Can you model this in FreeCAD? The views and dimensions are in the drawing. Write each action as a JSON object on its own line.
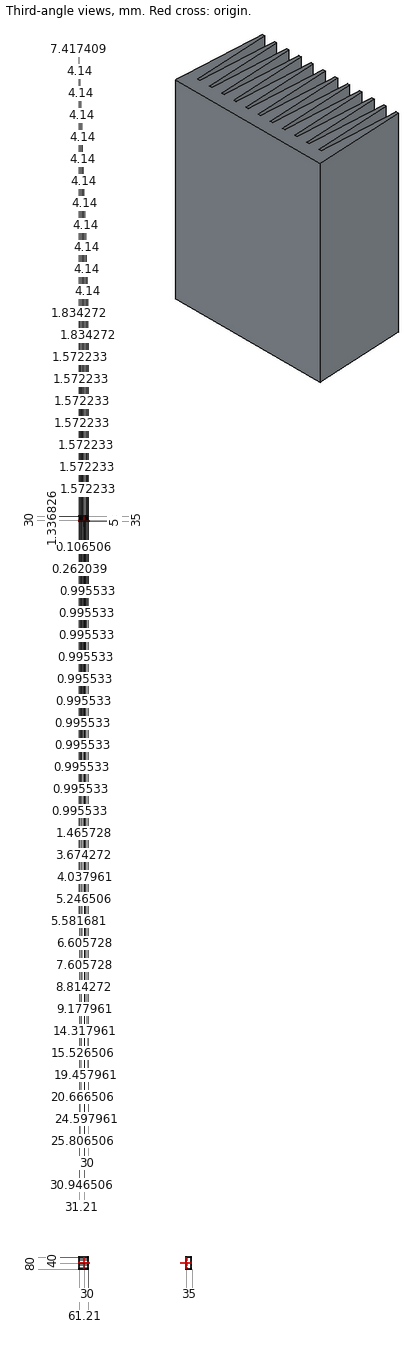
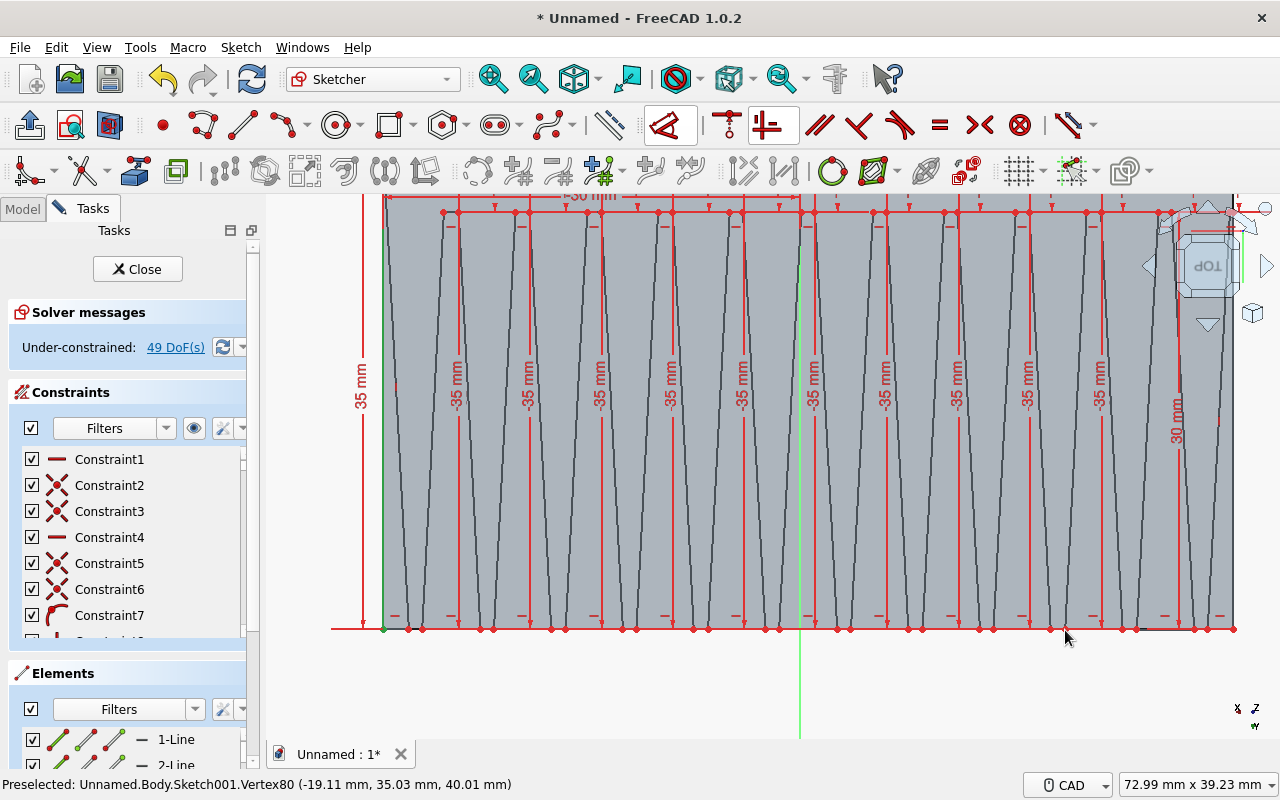
{"action": "scroll", "coordinate": [494, 630], "scroll_direction": "down", "scroll_amount": 2}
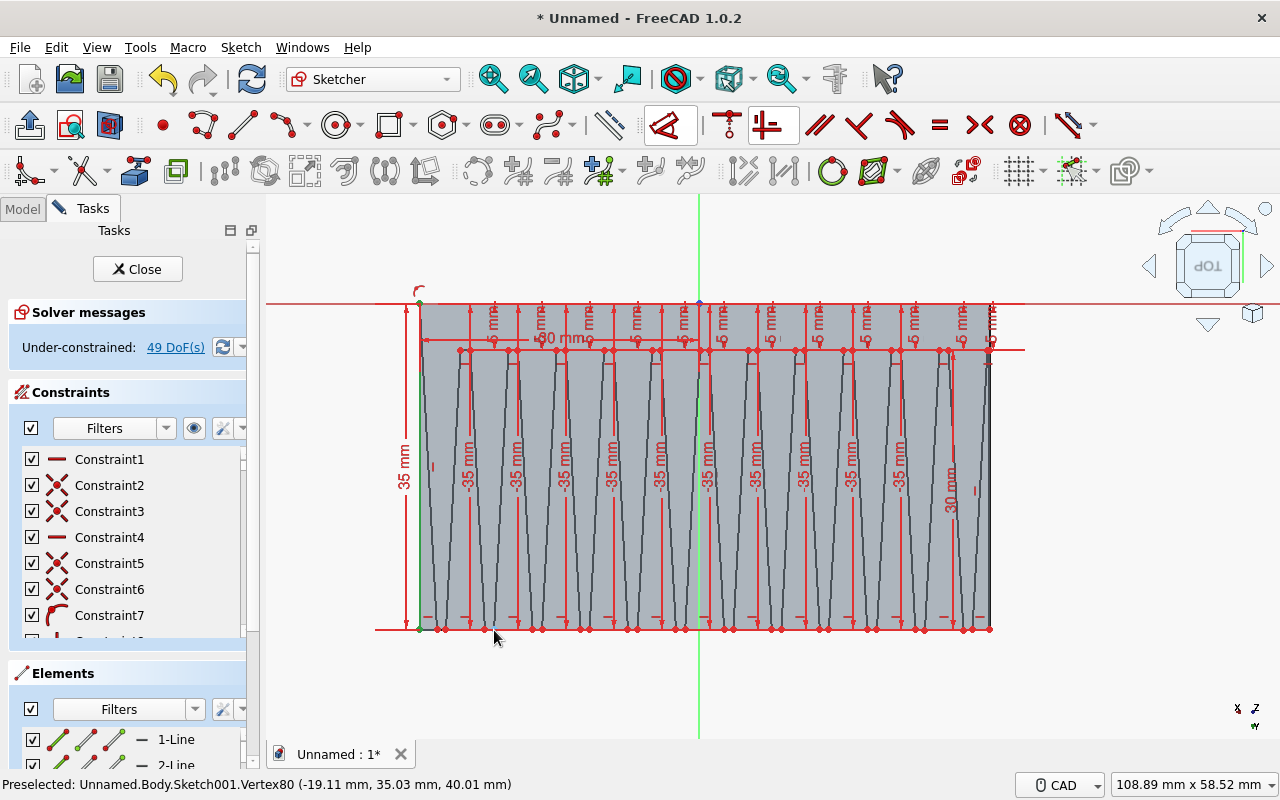
{"action": "scroll", "coordinate": [925, 630], "scroll_direction": "up", "scroll_amount": 2}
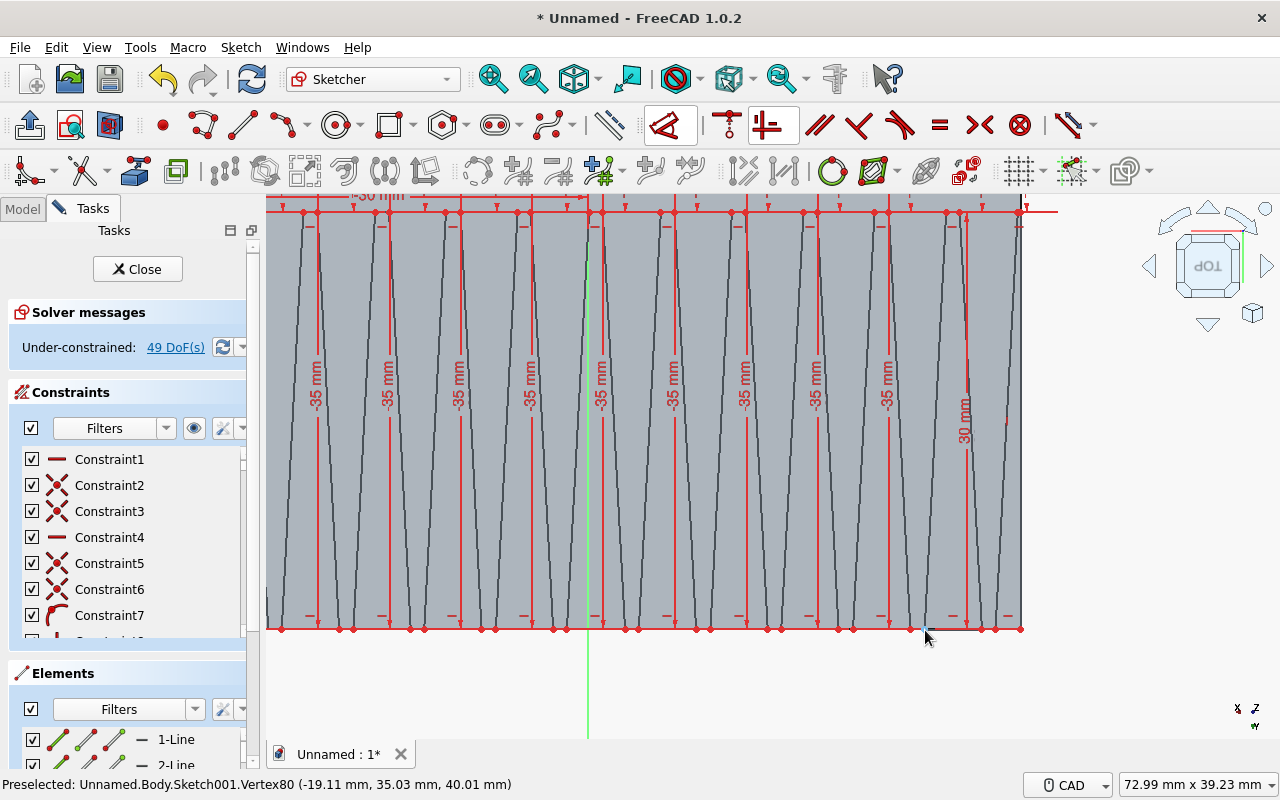
{"action": "left_click", "coordinate": [925, 630]}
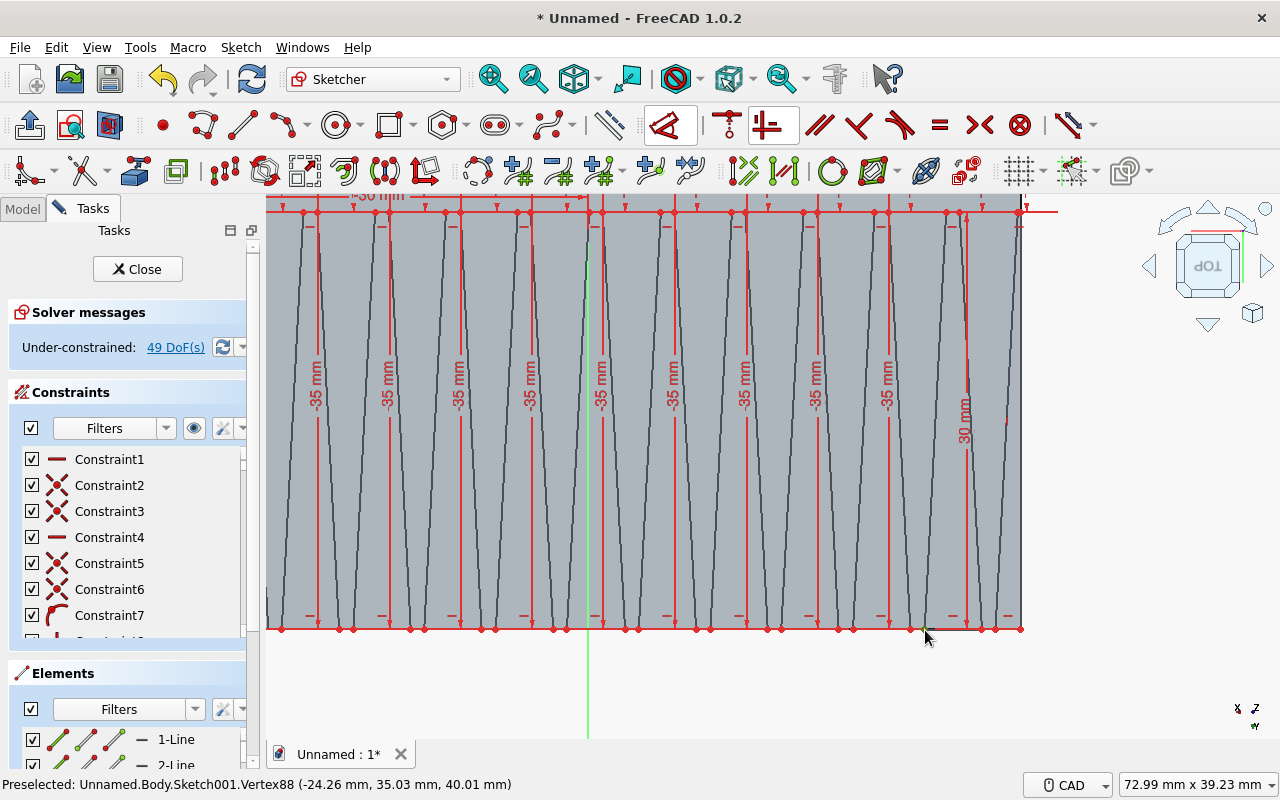
{"action": "key", "text": "i"}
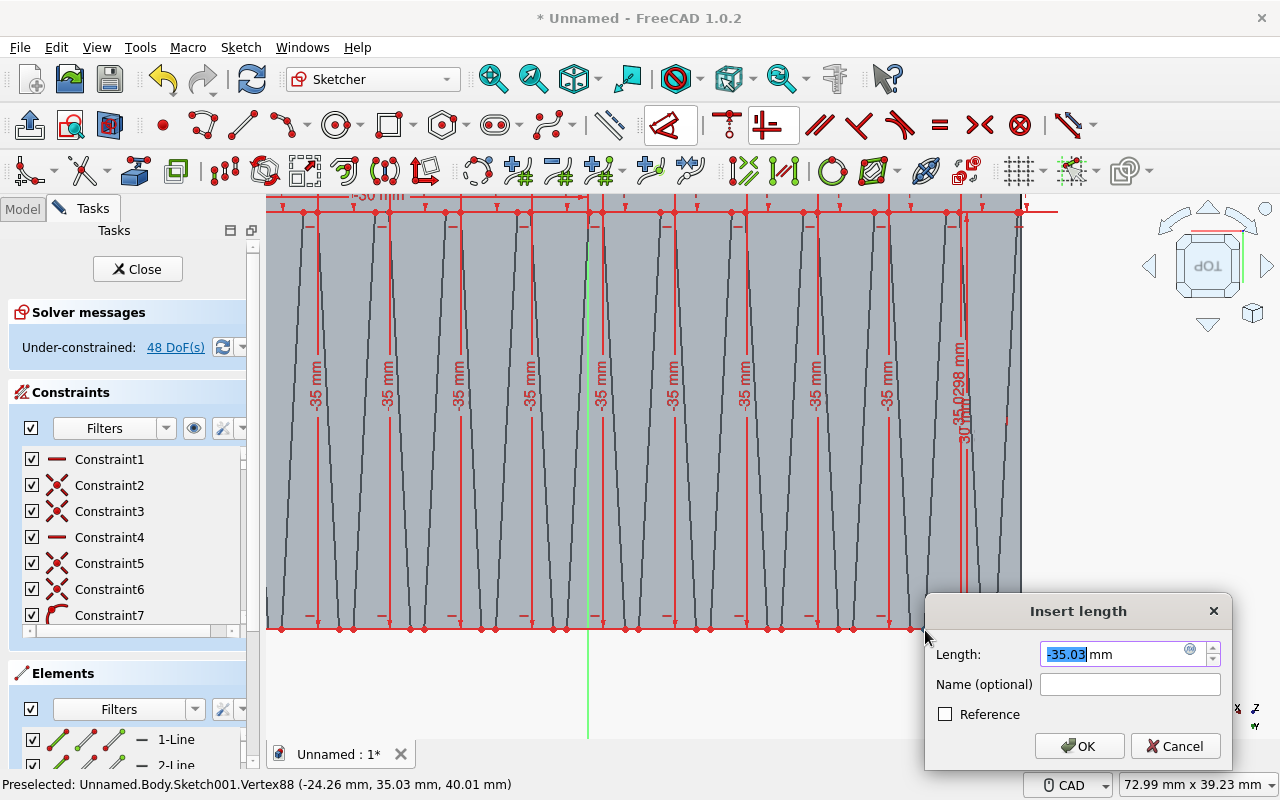
{"action": "type", "text": "-35"}
{"action": "key", "text": "Return"}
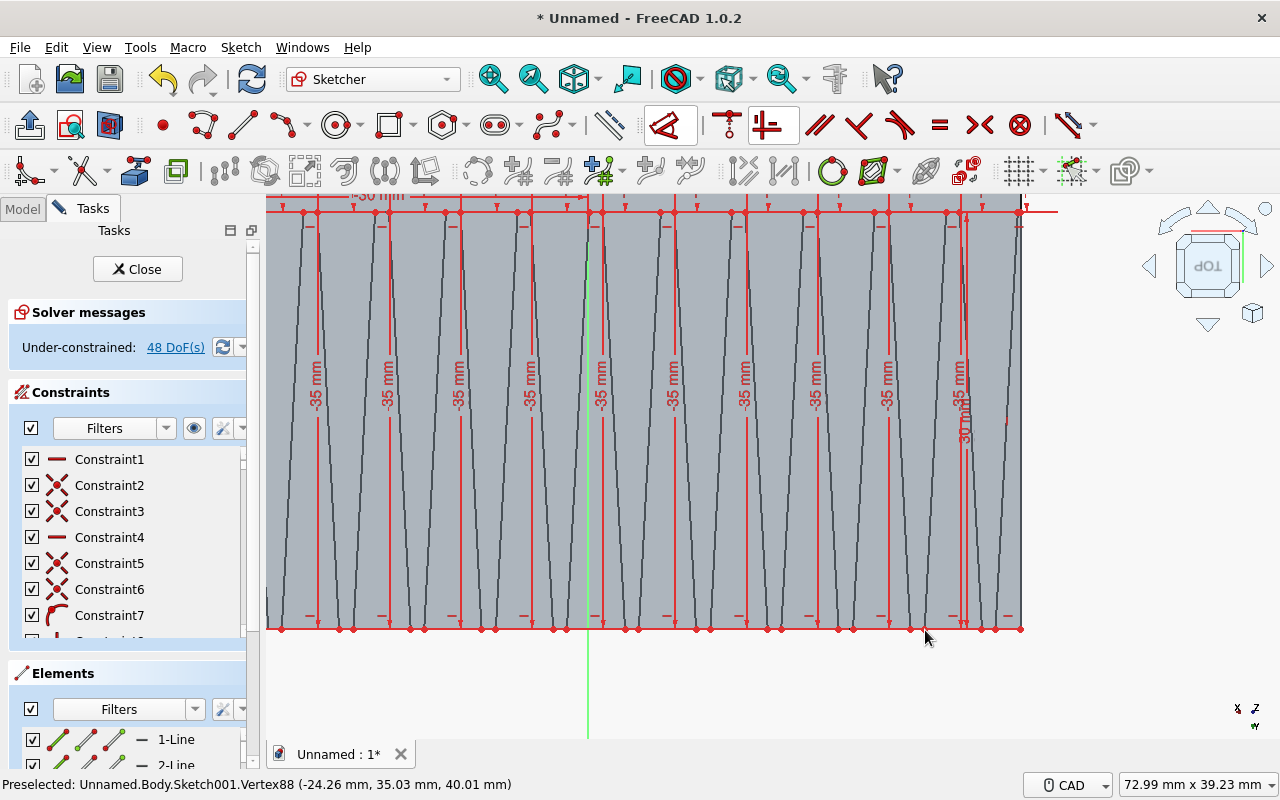
{"action": "scroll", "coordinate": [925, 630], "scroll_direction": "down", "scroll_amount": 2}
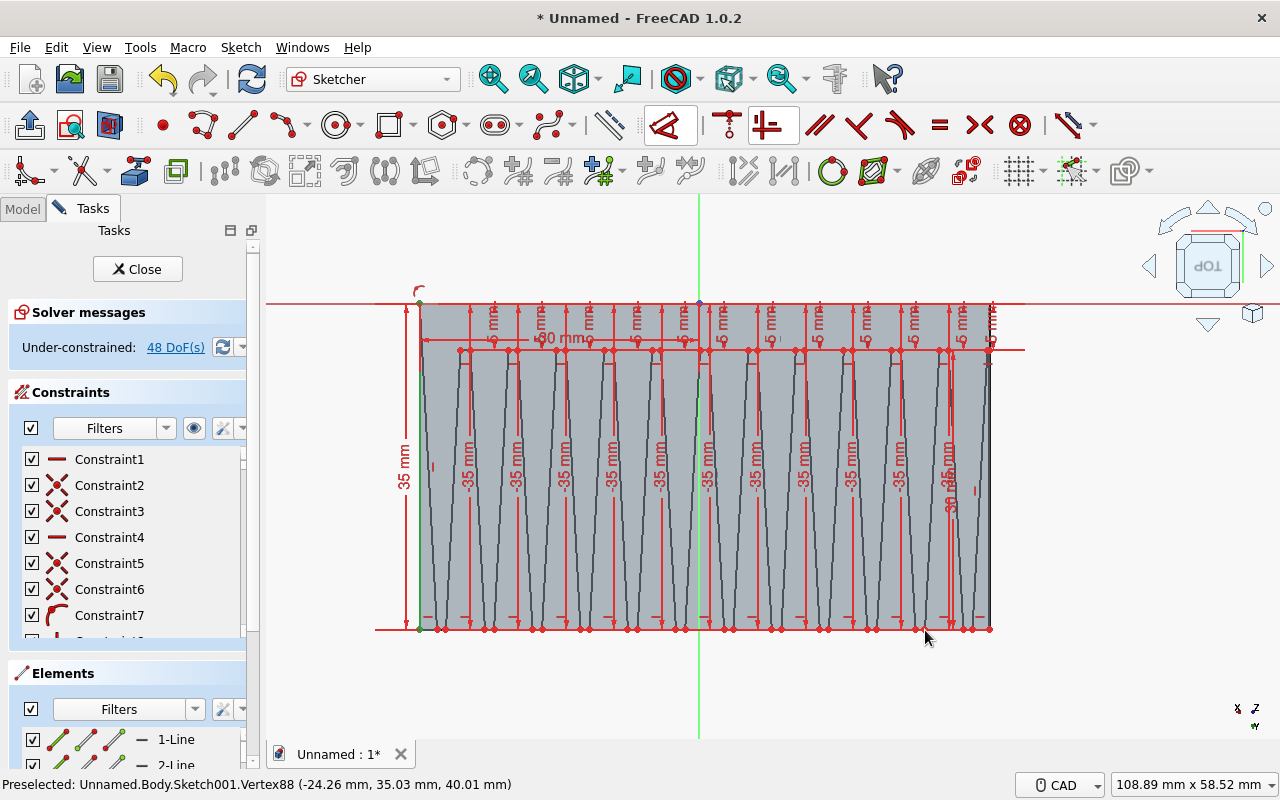
{"action": "left_click", "coordinate": [458, 630]}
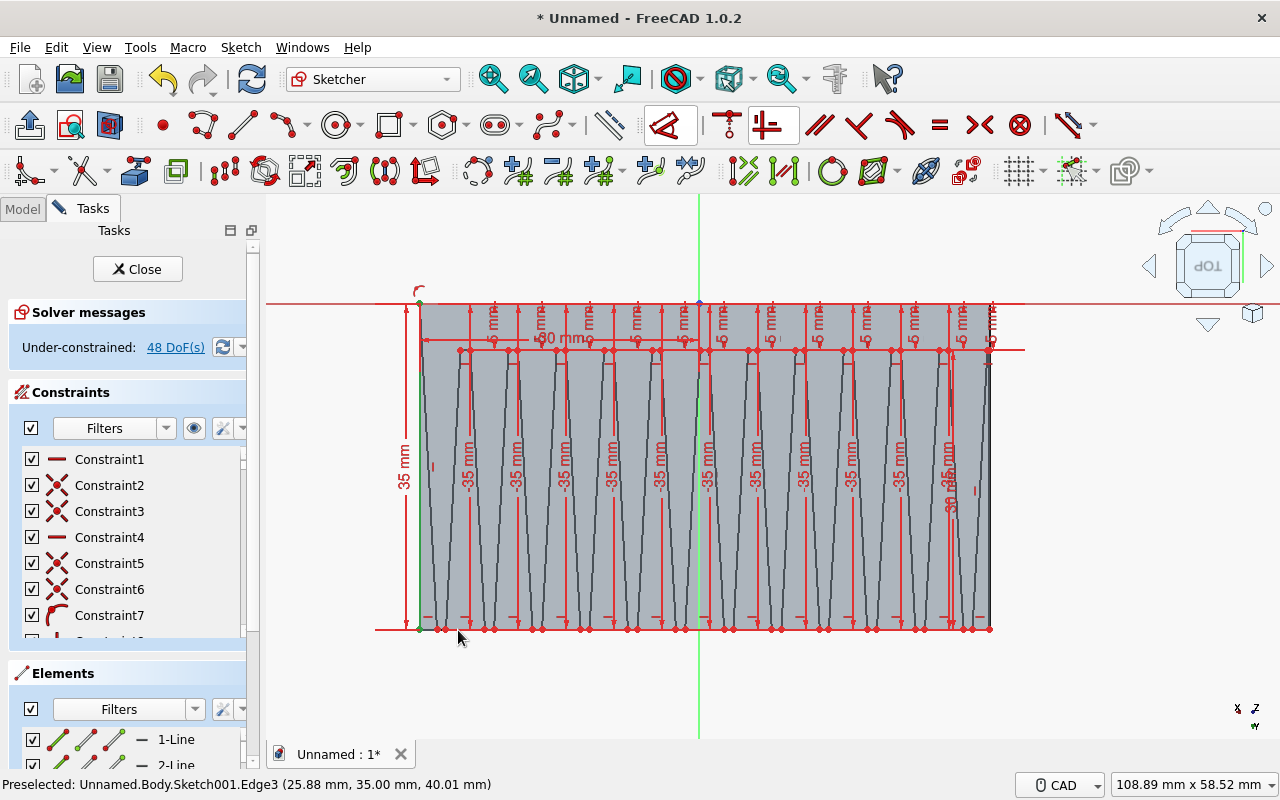
{"action": "key", "text": "l"}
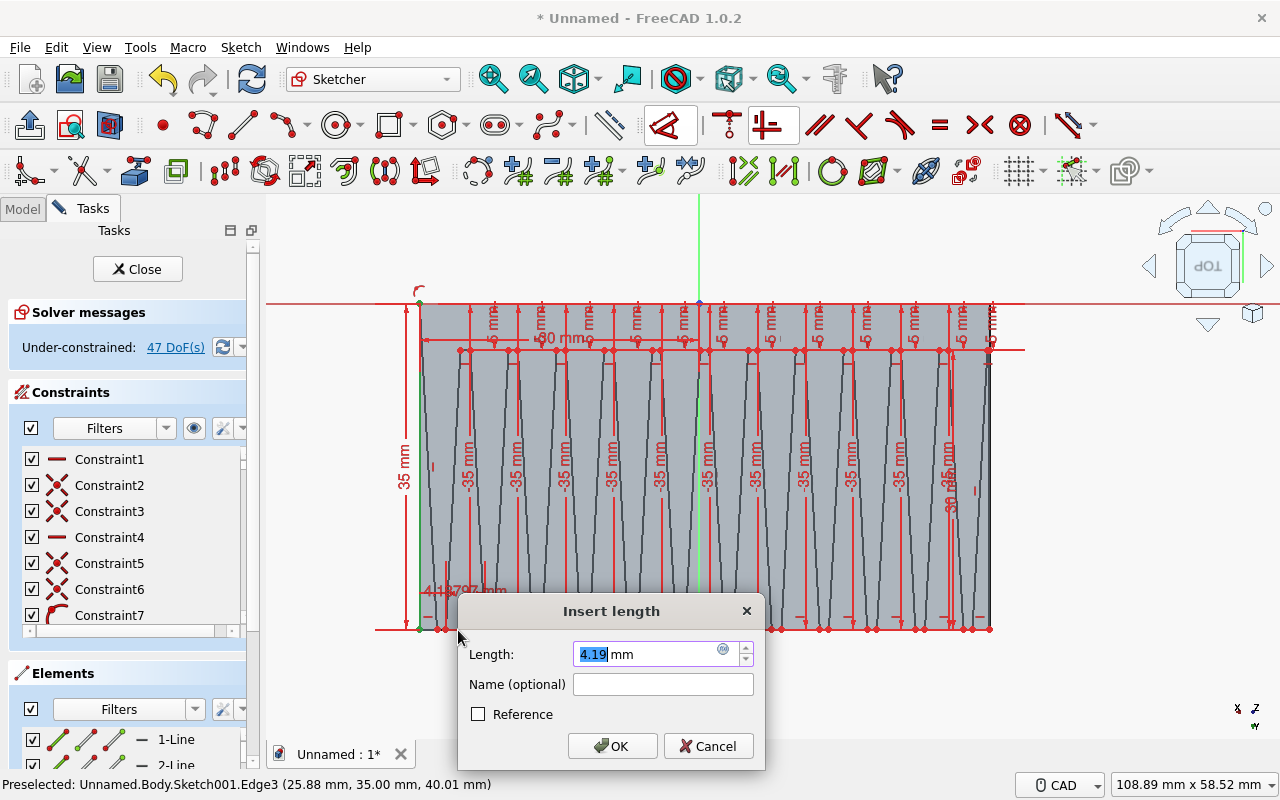
{"action": "type", "text": "4.14"}
{"action": "key", "text": "Return"}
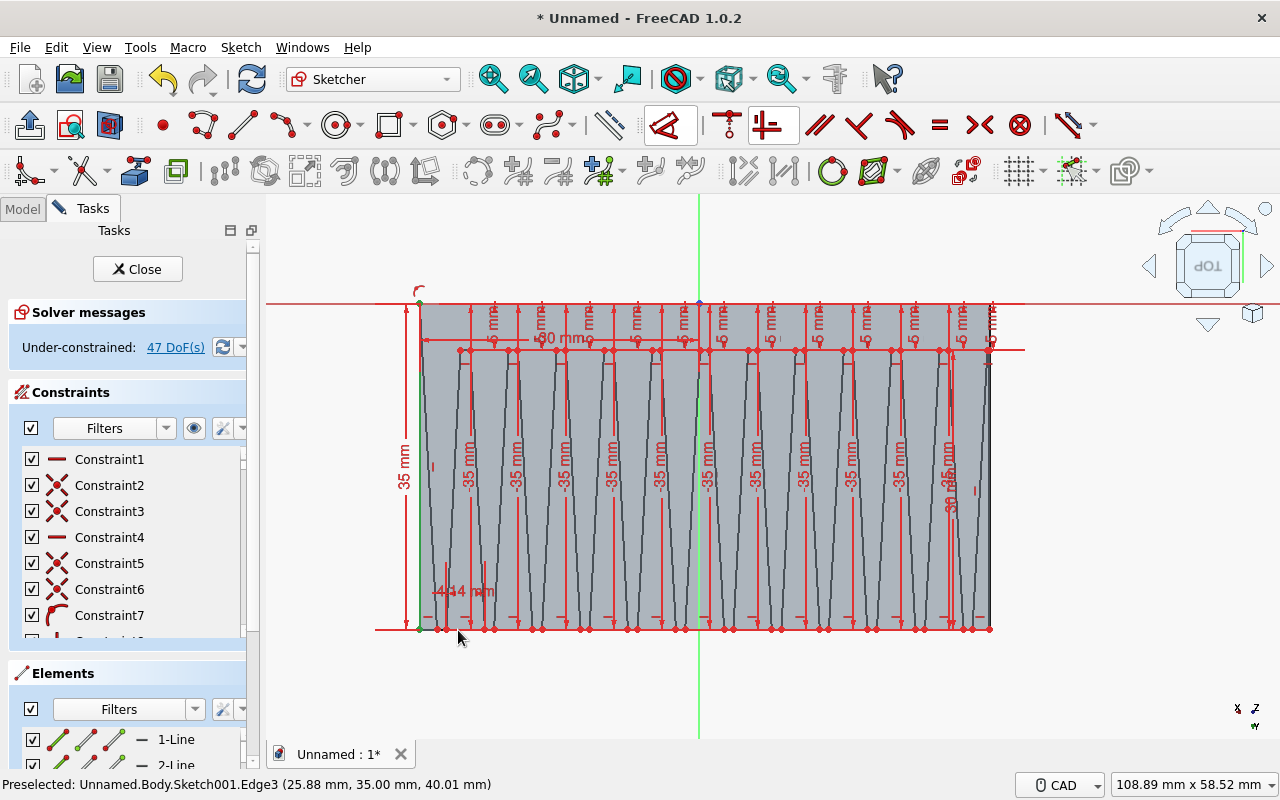
{"action": "left_click", "coordinate": [506, 630]}